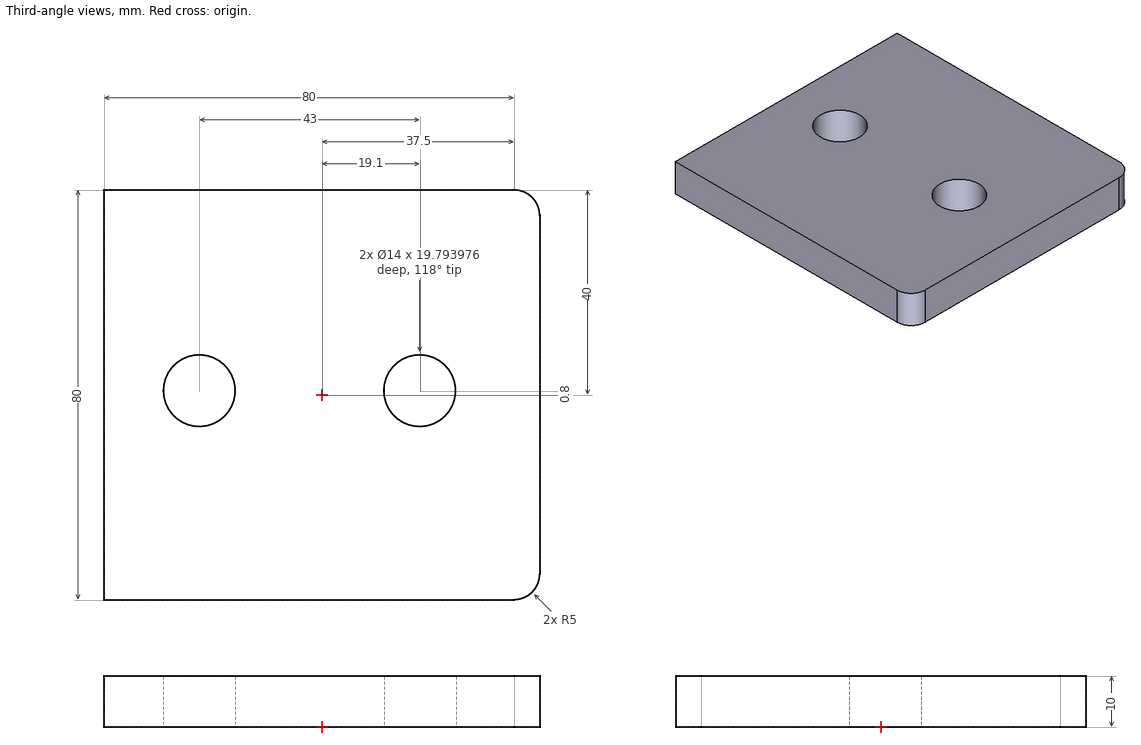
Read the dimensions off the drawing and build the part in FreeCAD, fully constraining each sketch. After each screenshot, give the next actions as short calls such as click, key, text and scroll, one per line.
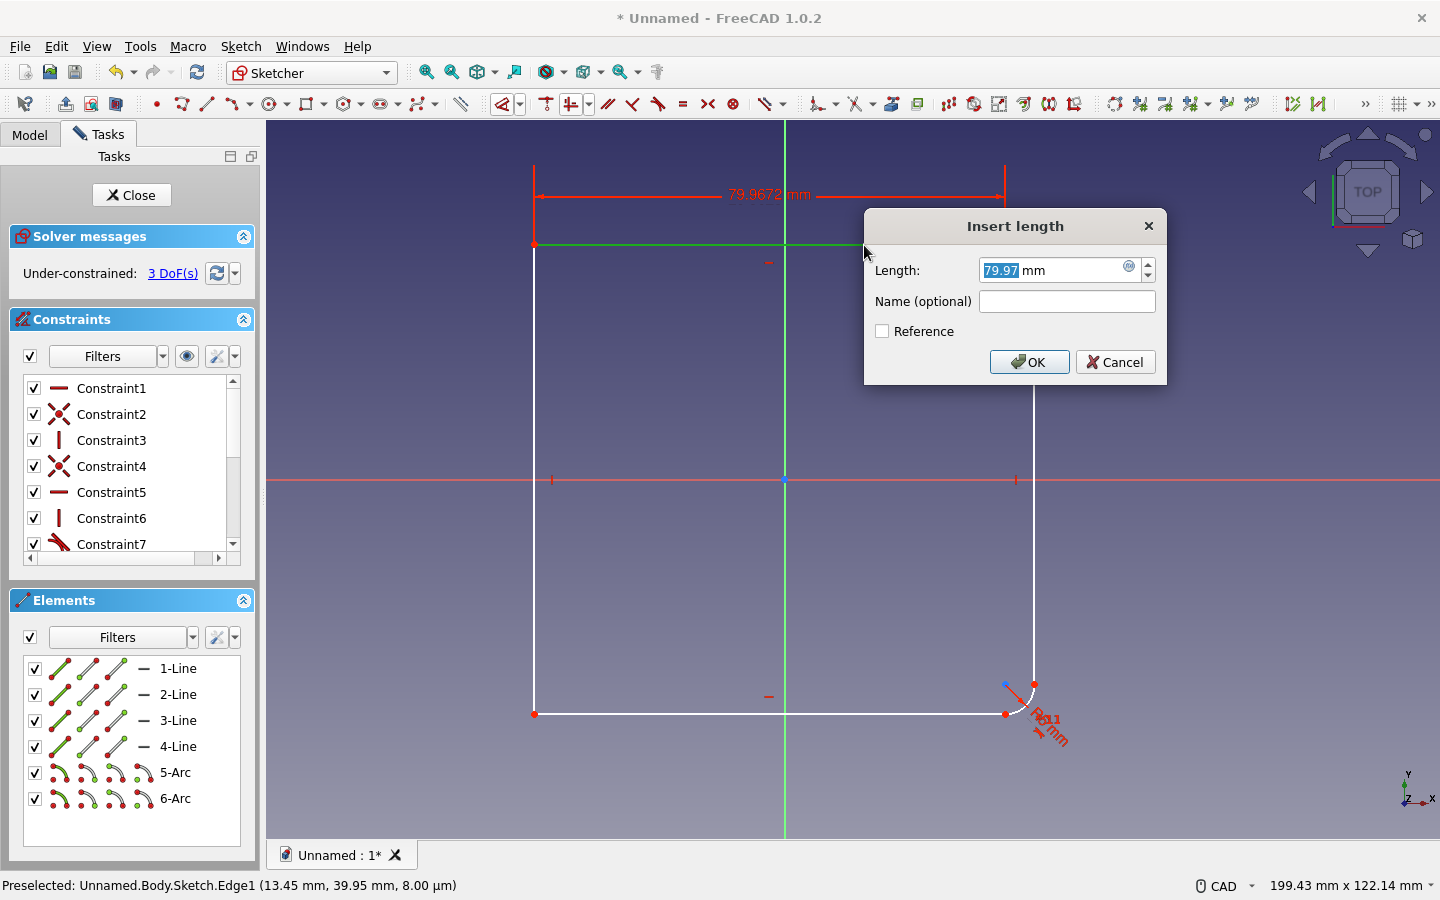
text(80)
key(Return)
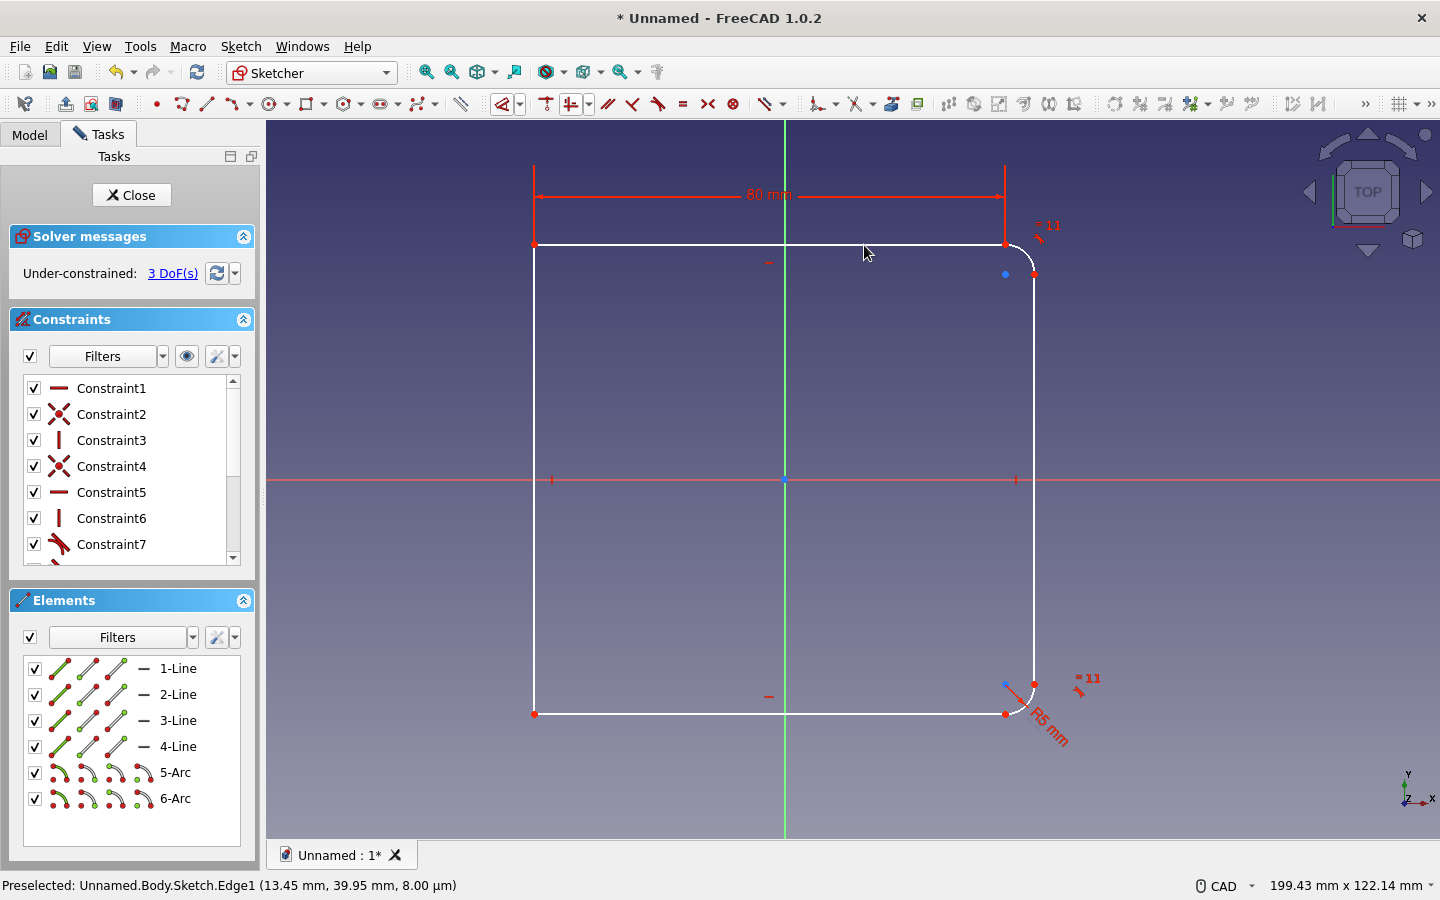
click(534, 386)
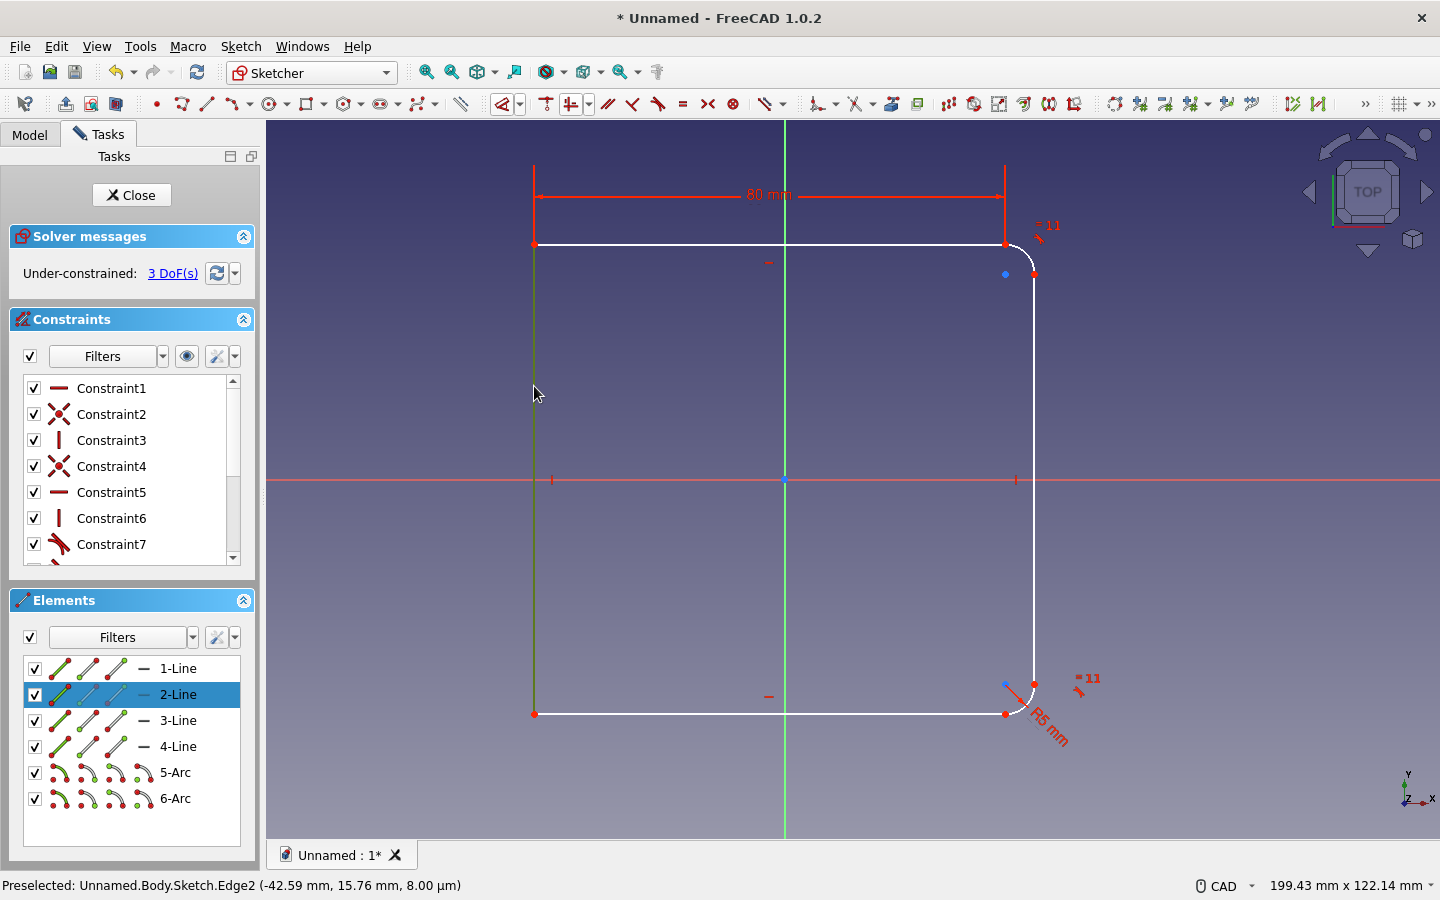
key(i)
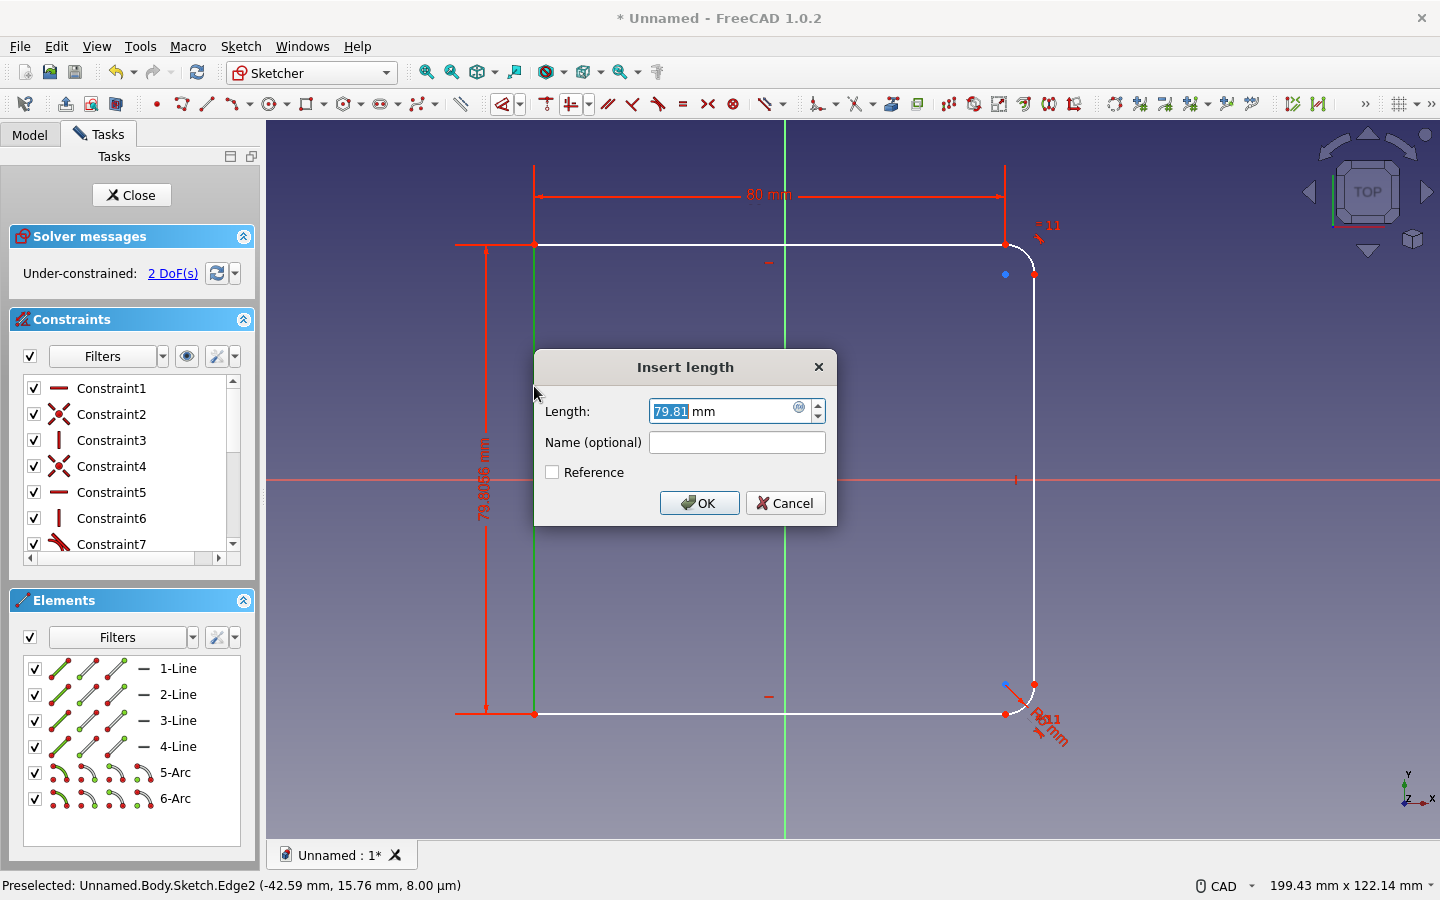
text(80)
key(Return)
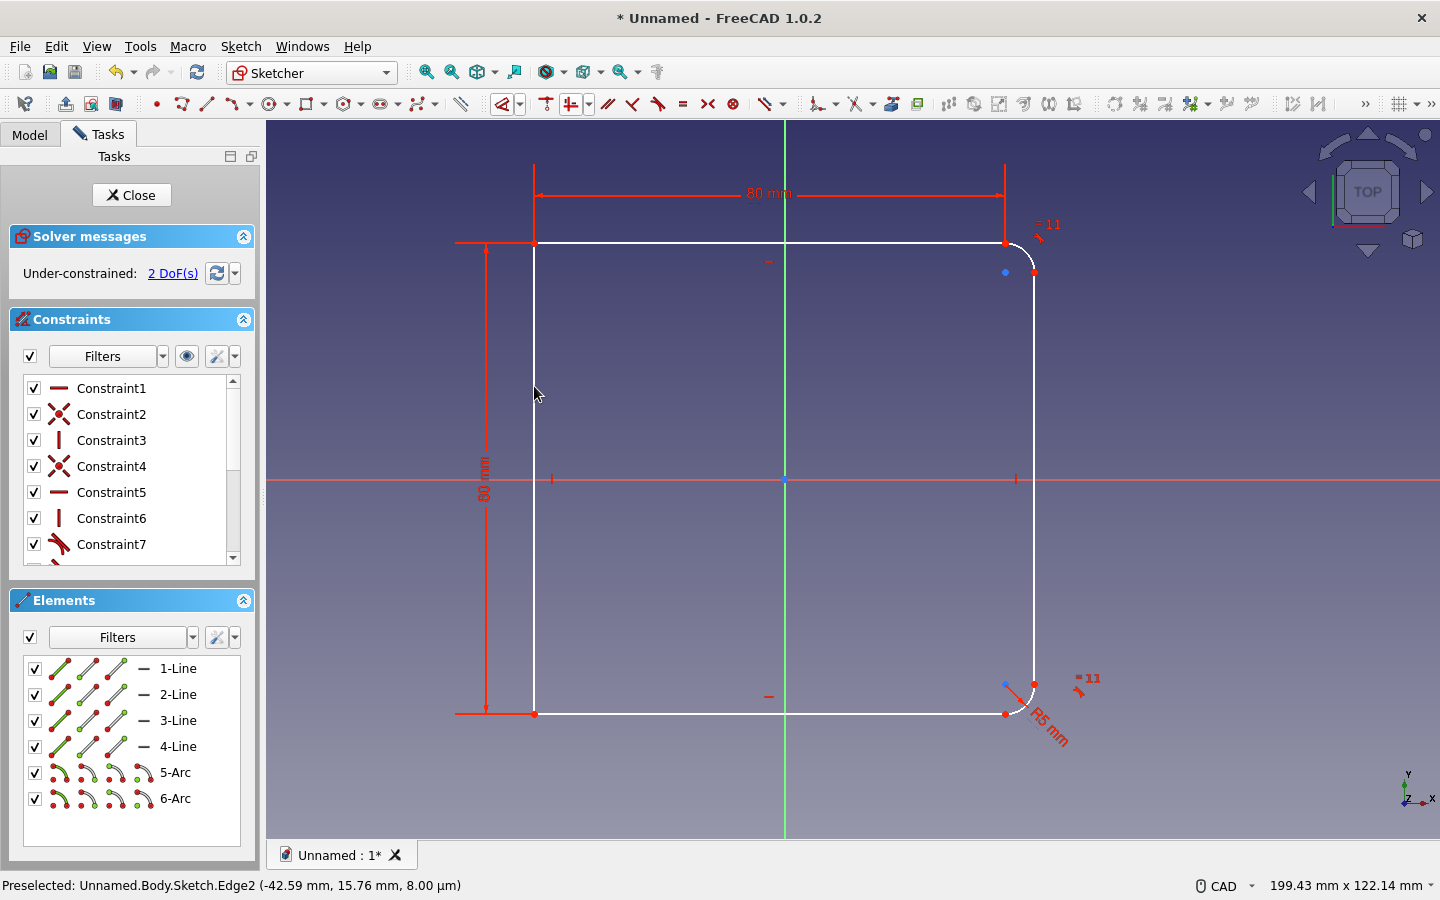
click(1005, 243)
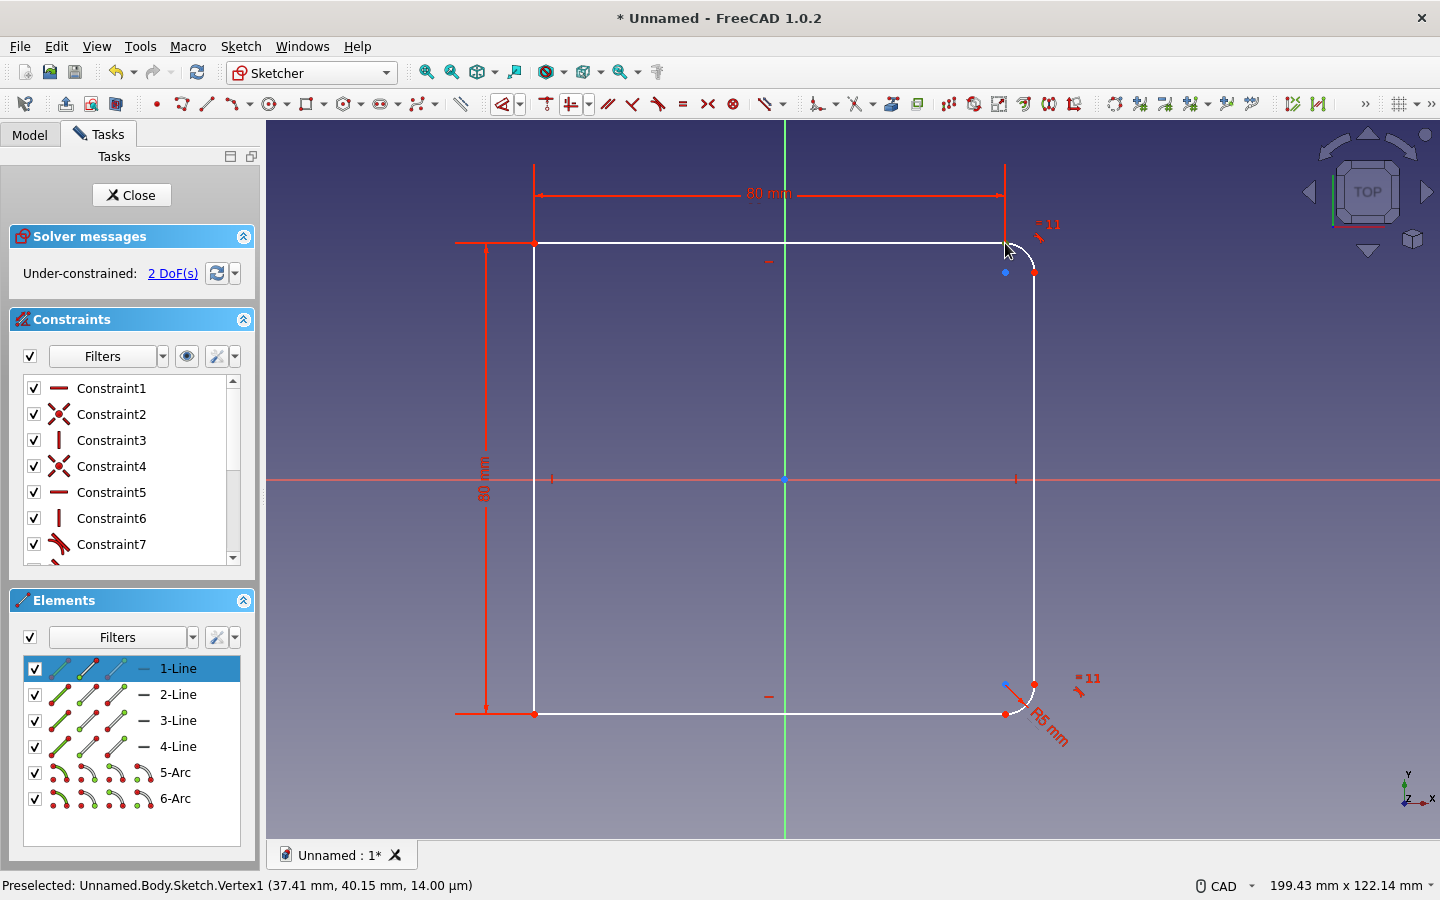
key(i)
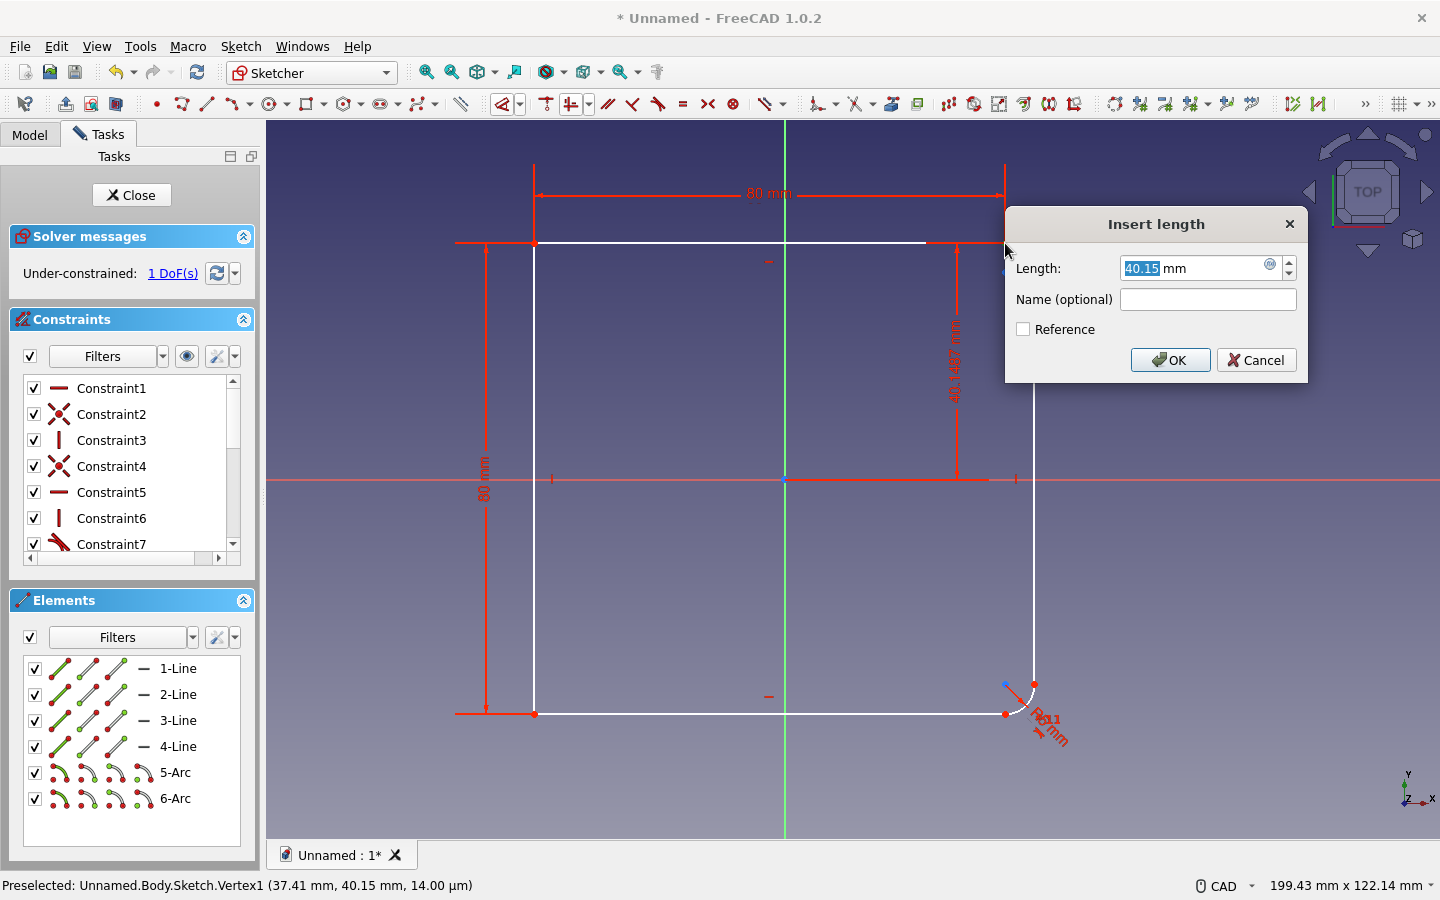
text(40)
key(Return)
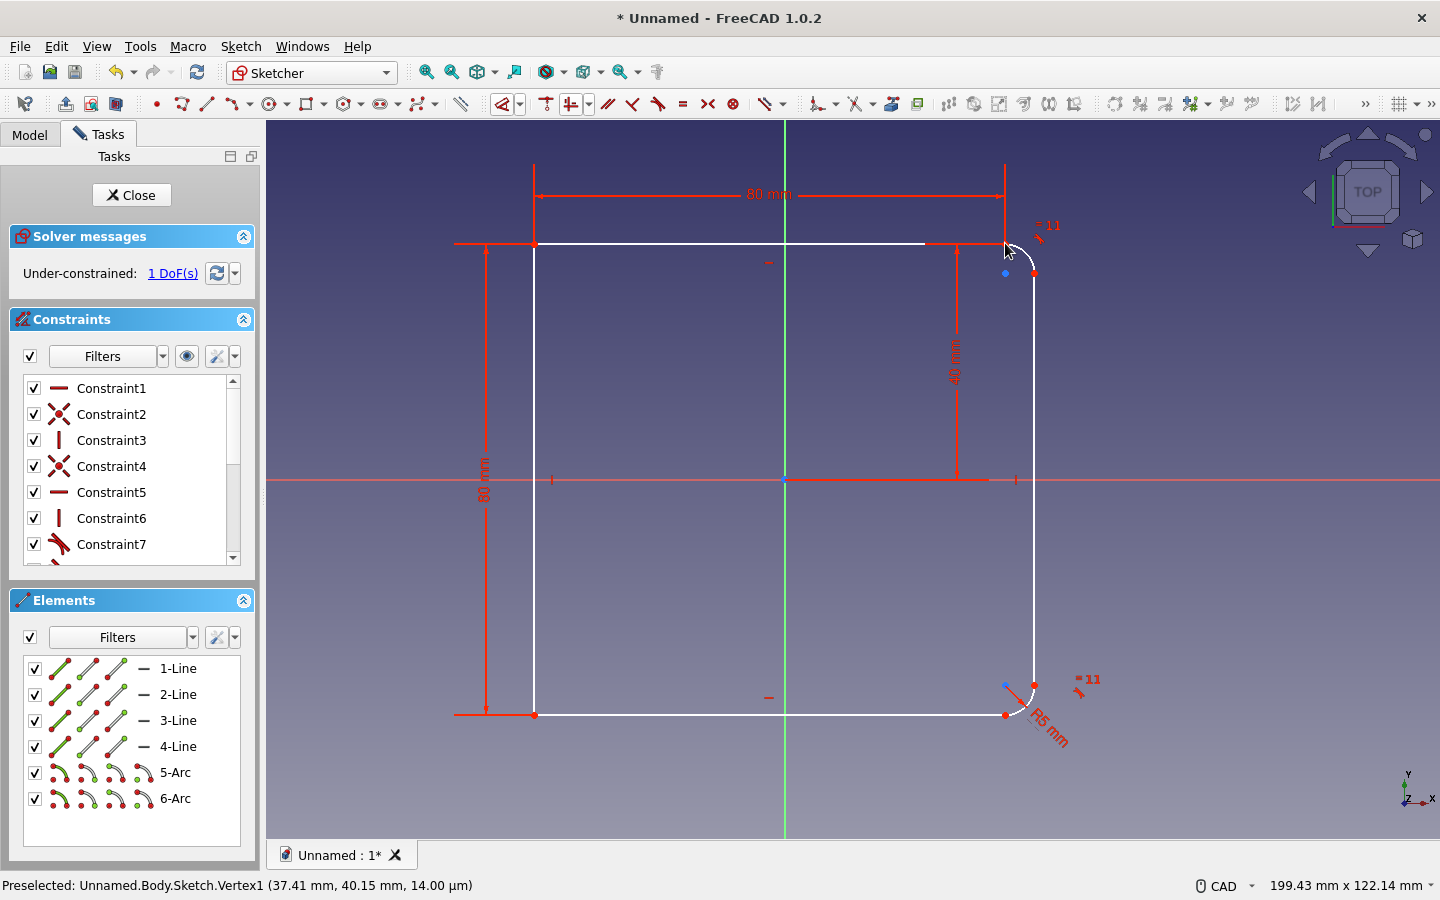
click(1005, 244)